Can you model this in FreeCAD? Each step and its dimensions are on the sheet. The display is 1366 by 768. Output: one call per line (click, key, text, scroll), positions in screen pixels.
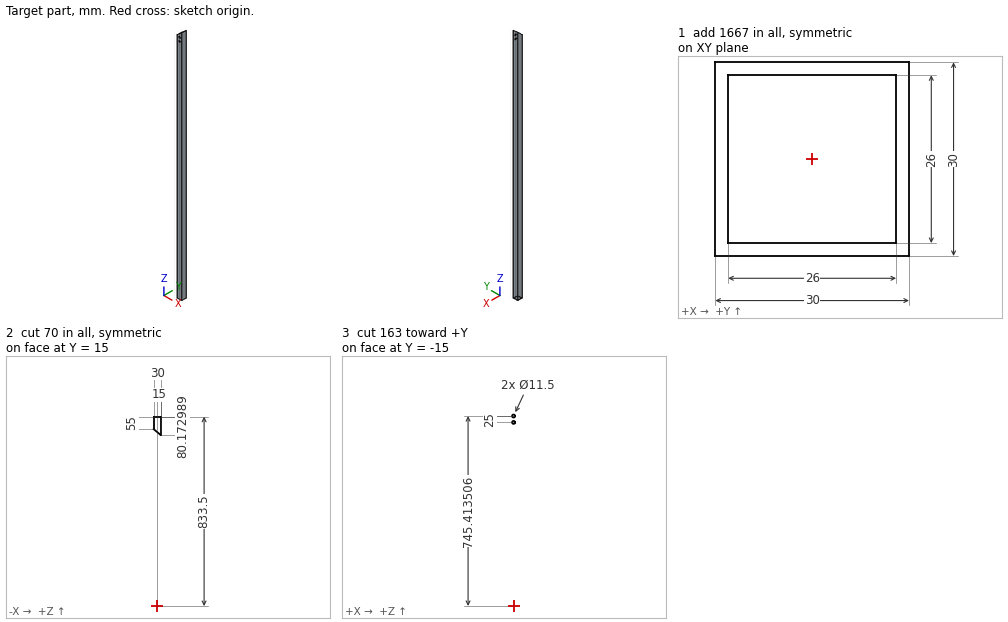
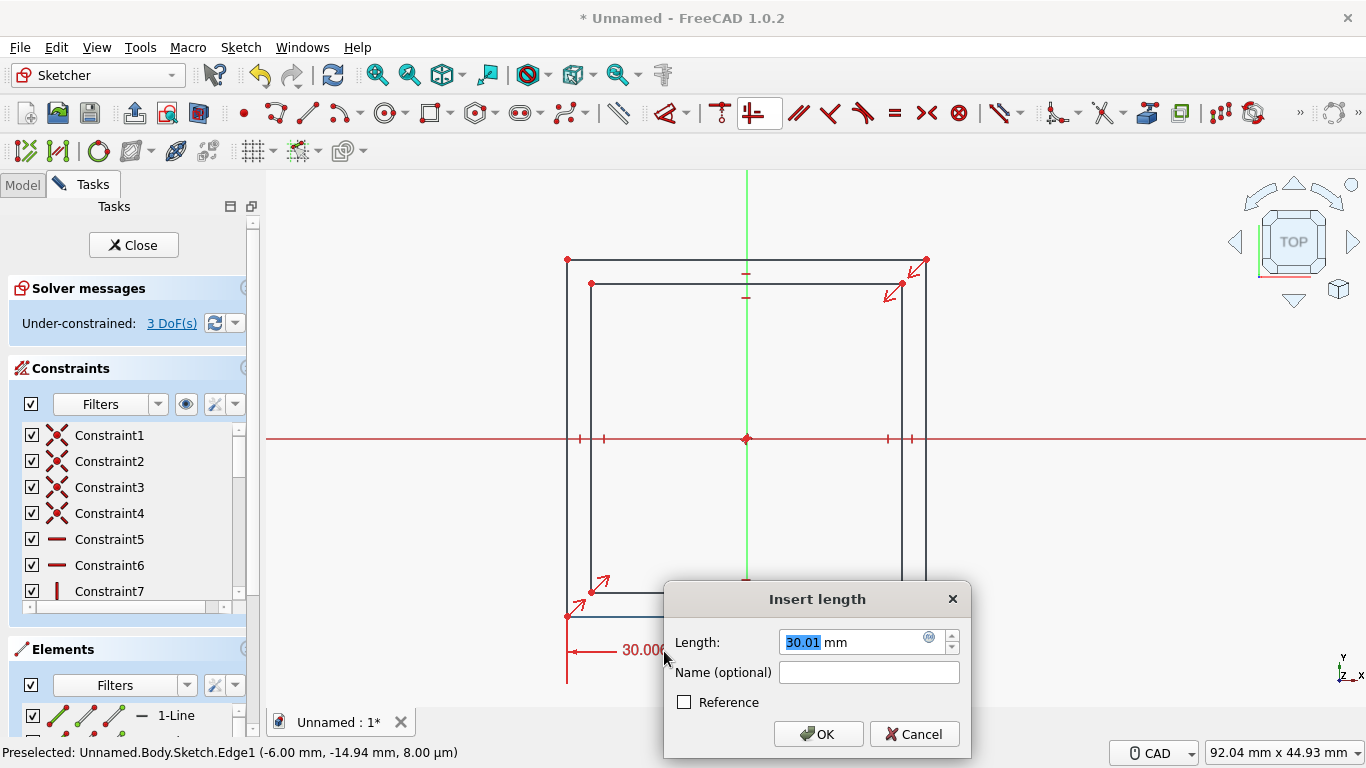
text(30)
key(Return)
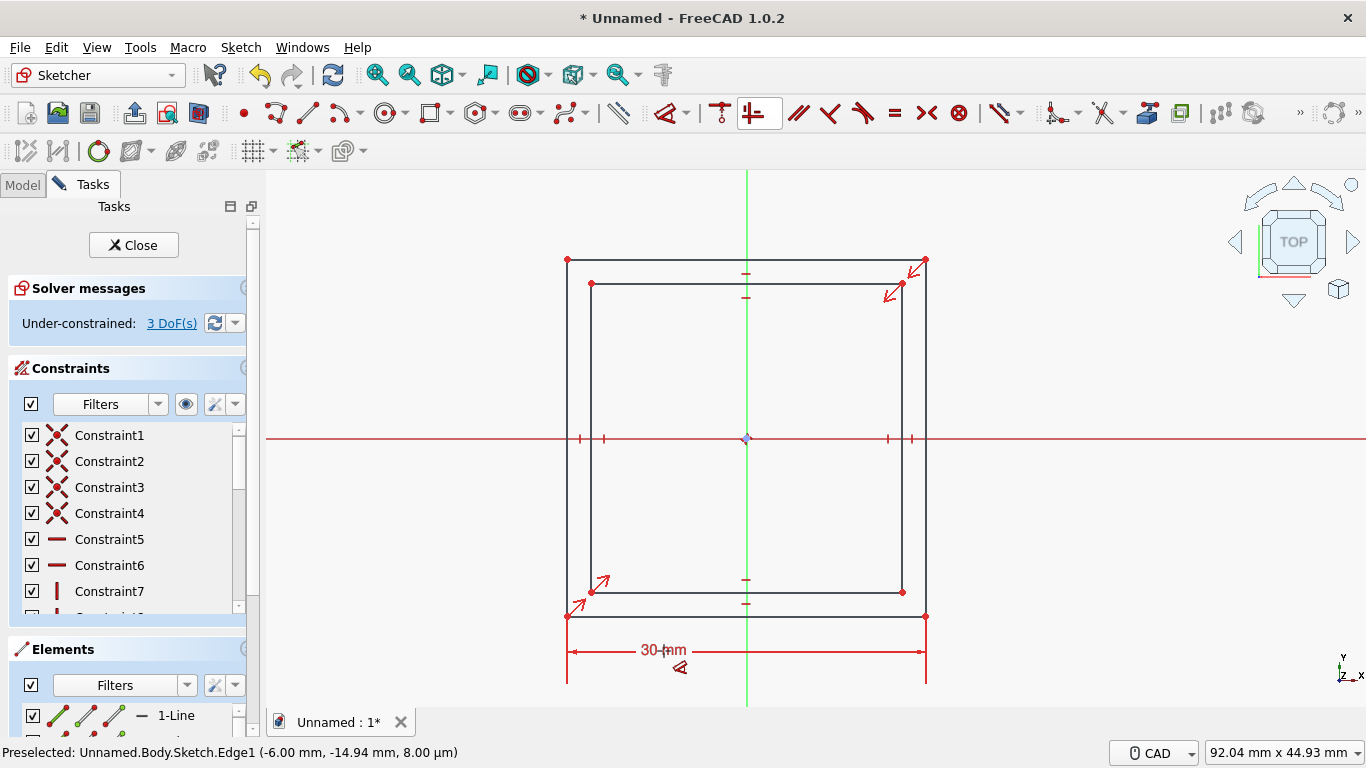
click(926, 510)
click(960, 356)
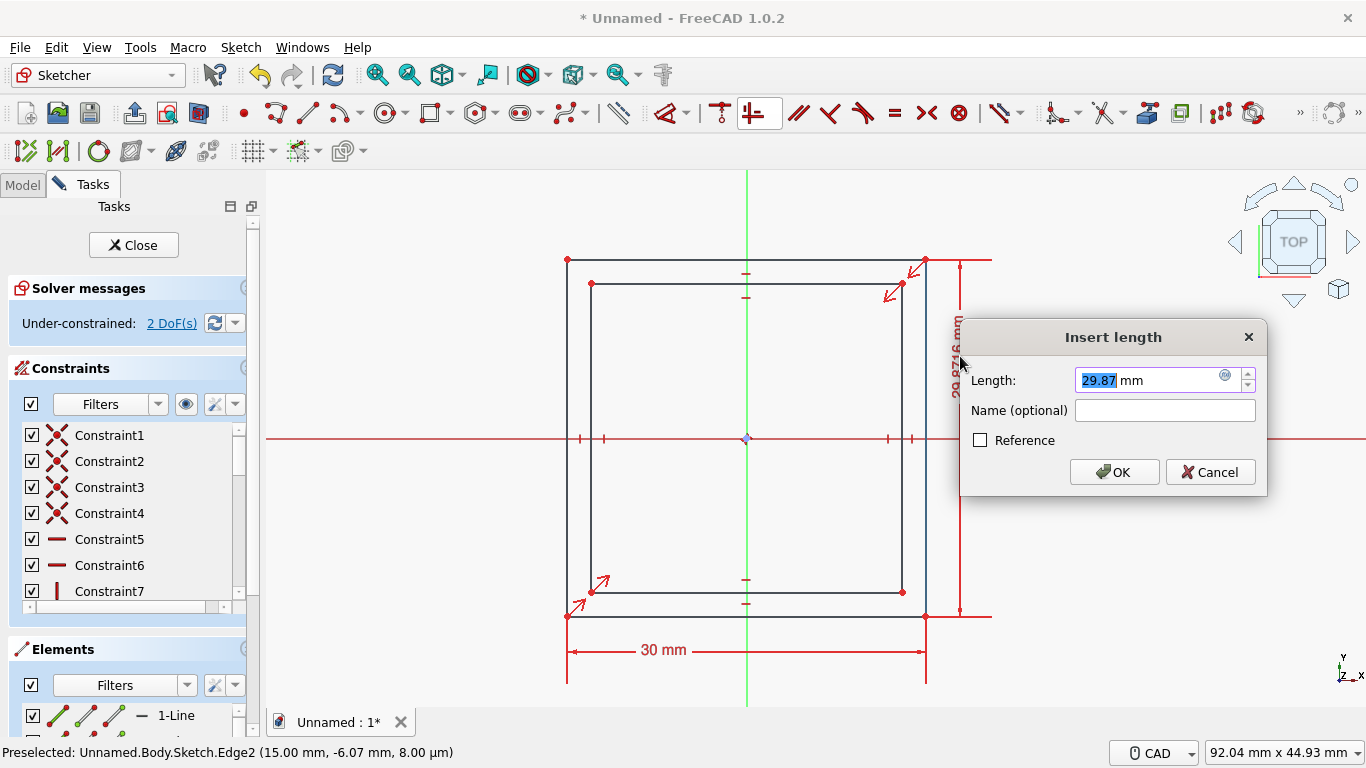
text(30)
key(Return)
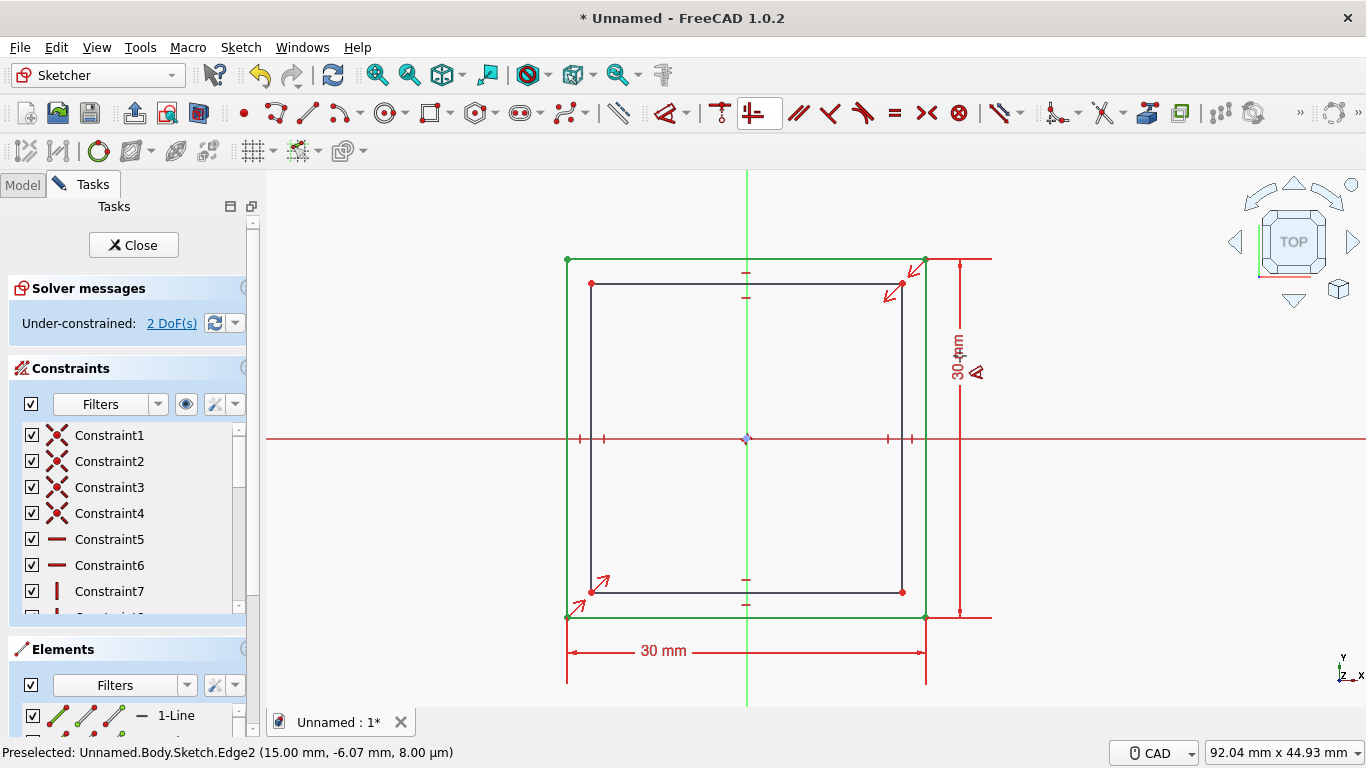
click(685, 593)
click(675, 559)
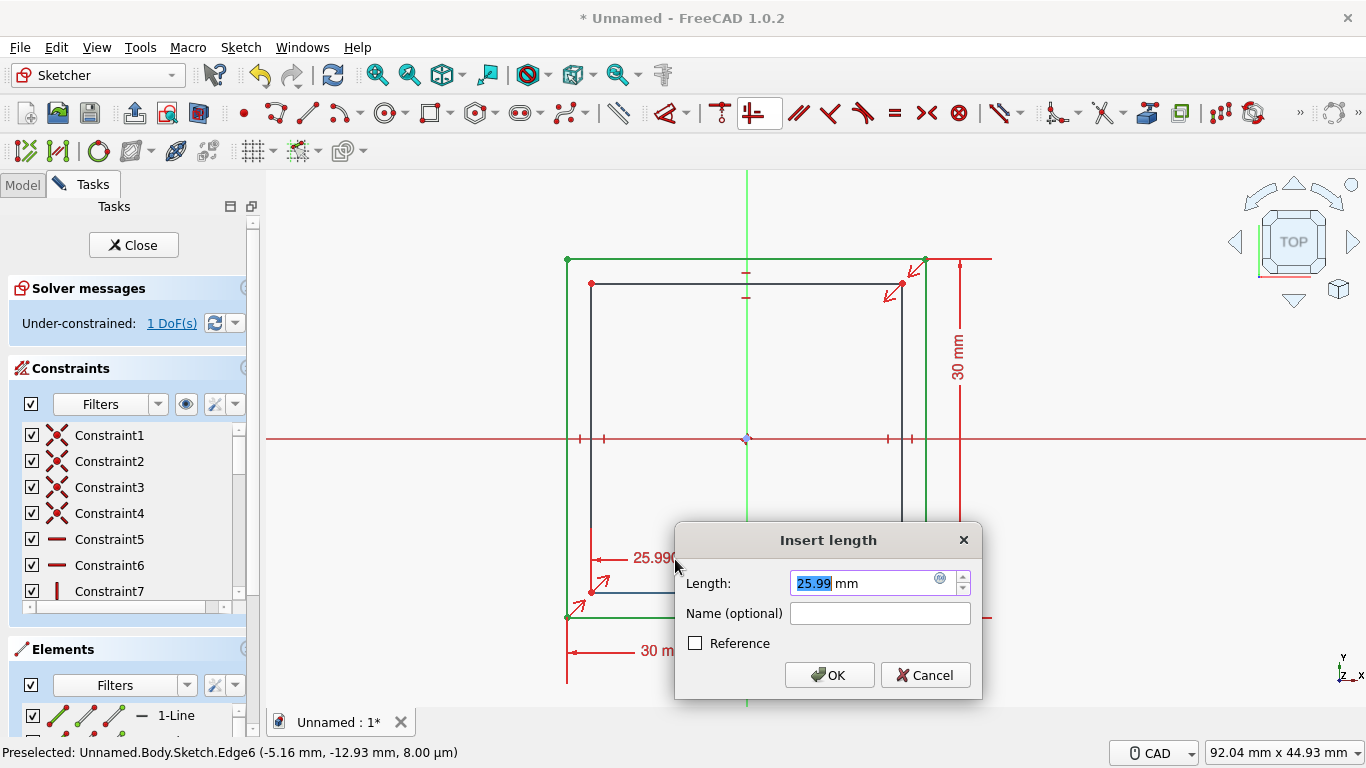
text(26)
key(Return)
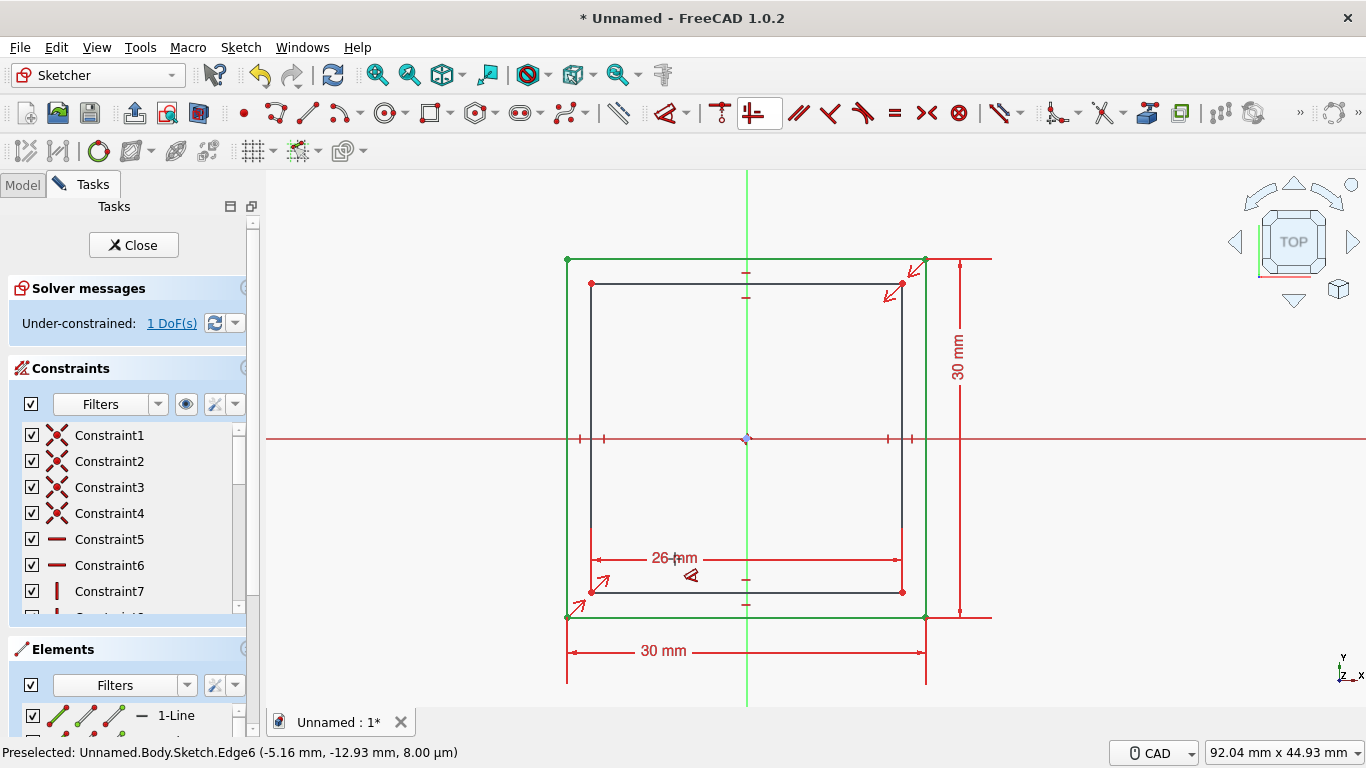
click(902, 500)
click(868, 367)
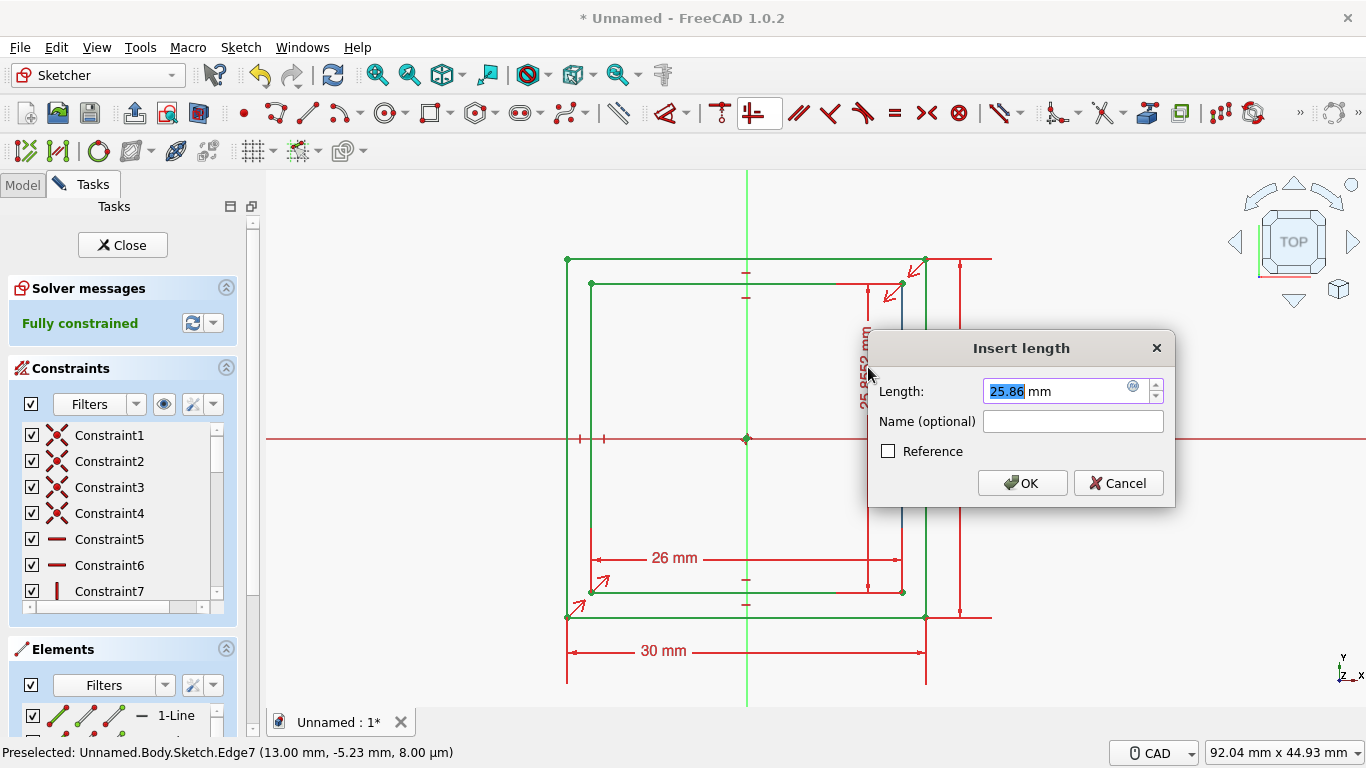
text(26)
key(Return)
key(Escape)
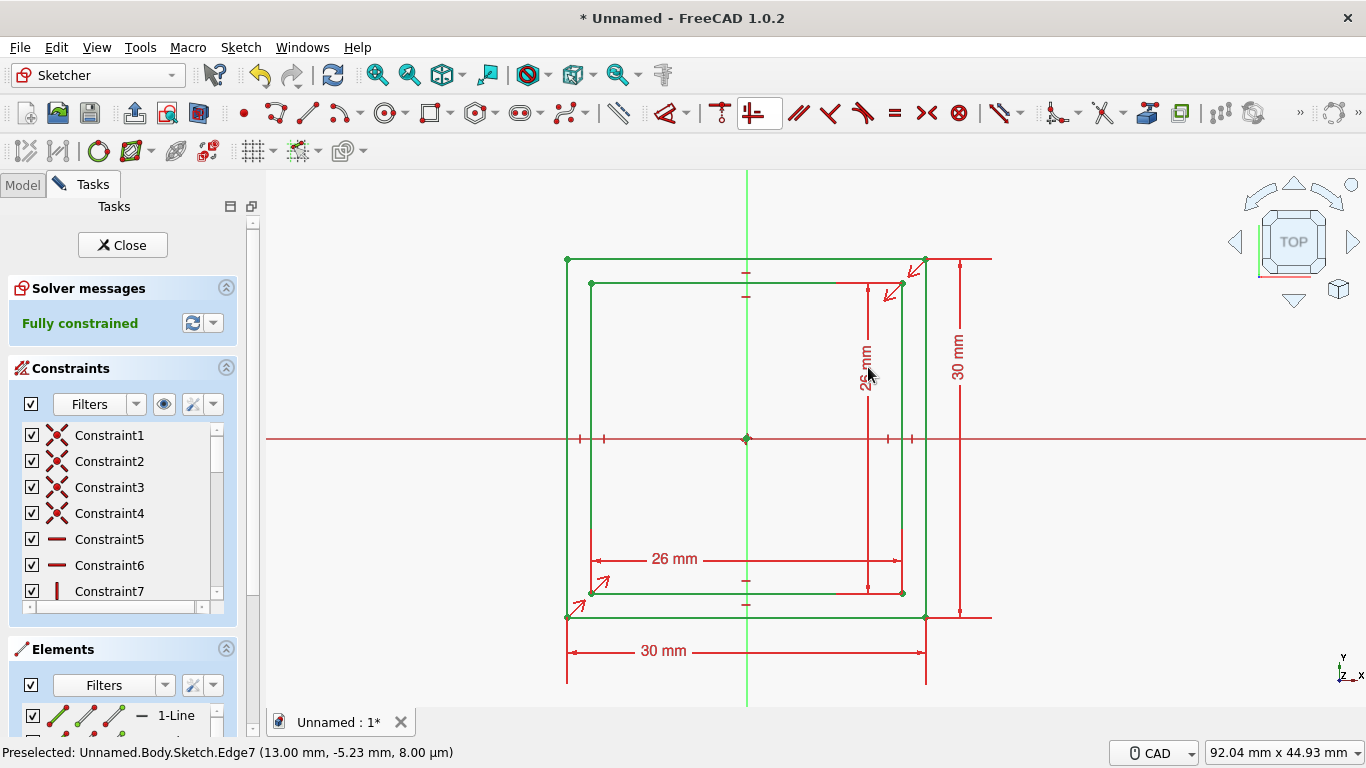
click(123, 245)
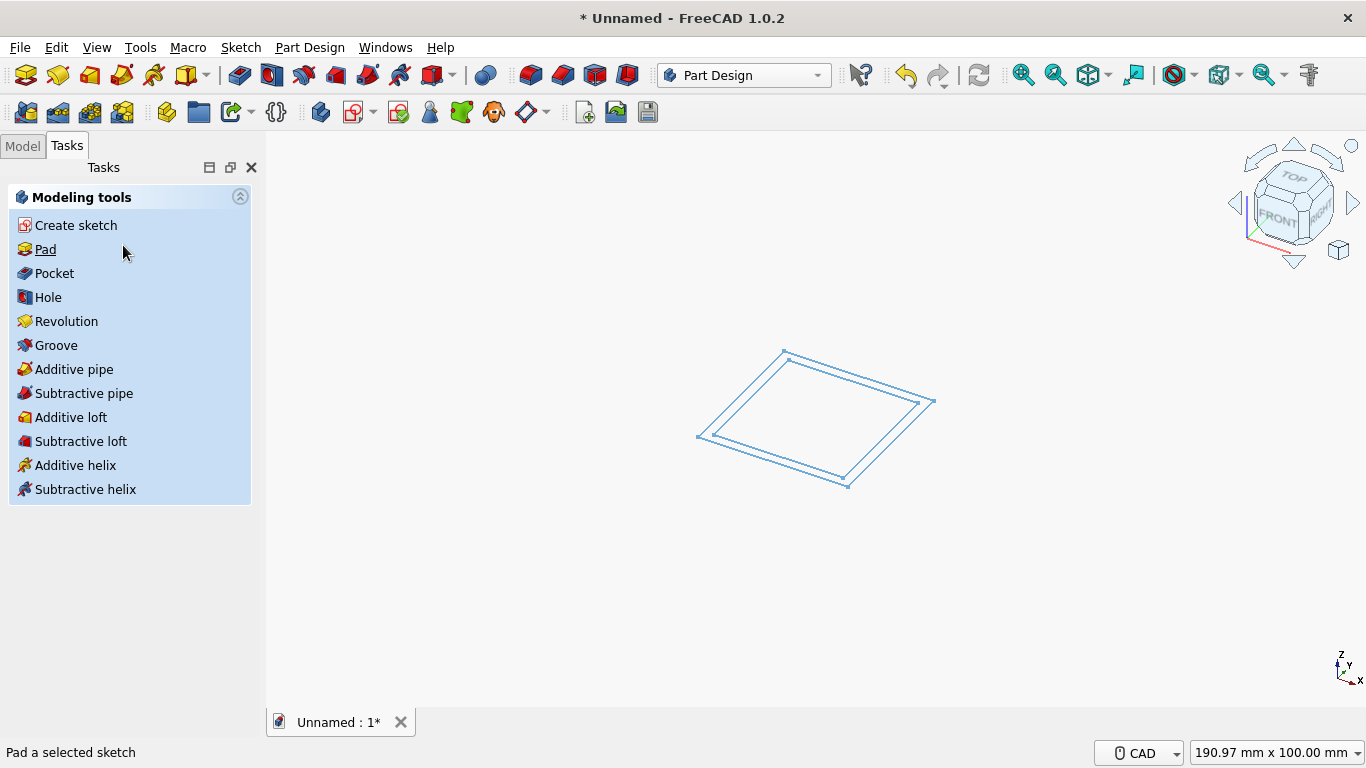
click(26, 76)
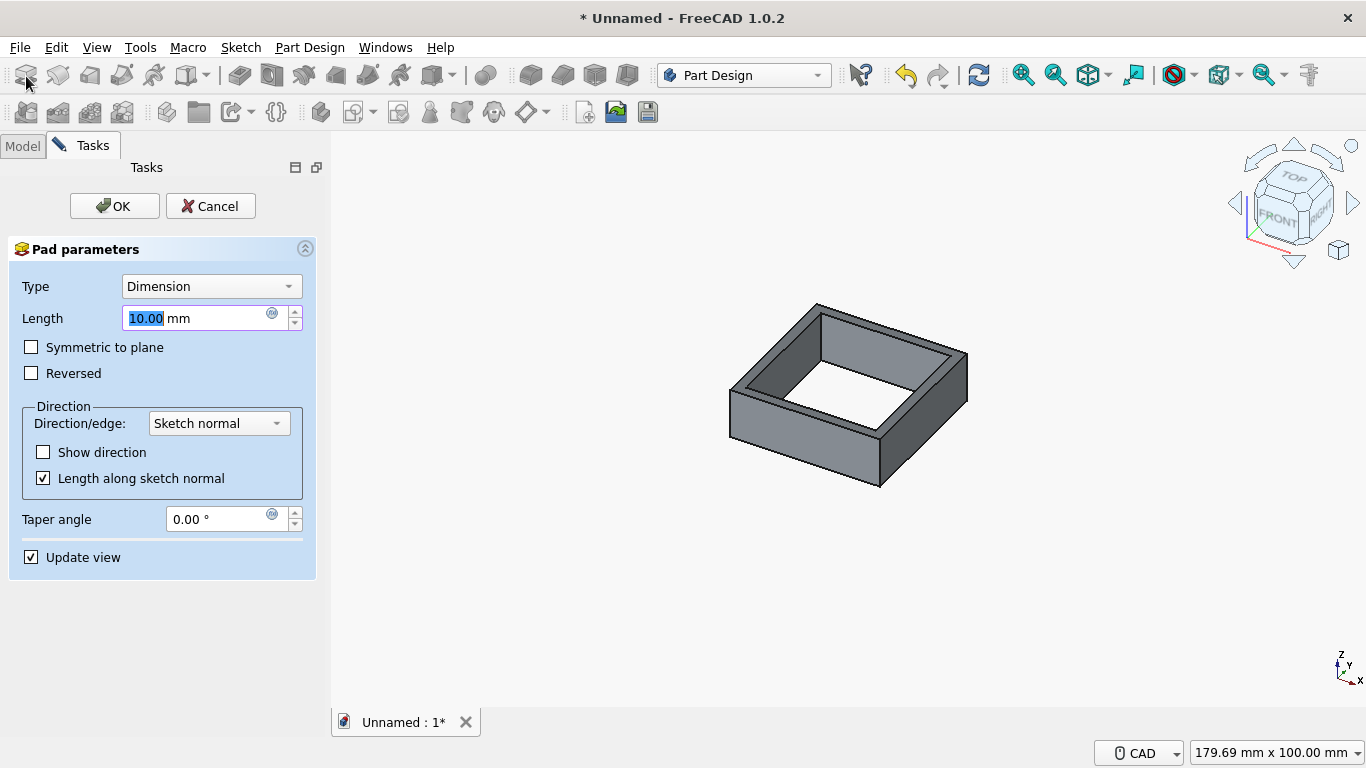
text(1667)
key(Tab)